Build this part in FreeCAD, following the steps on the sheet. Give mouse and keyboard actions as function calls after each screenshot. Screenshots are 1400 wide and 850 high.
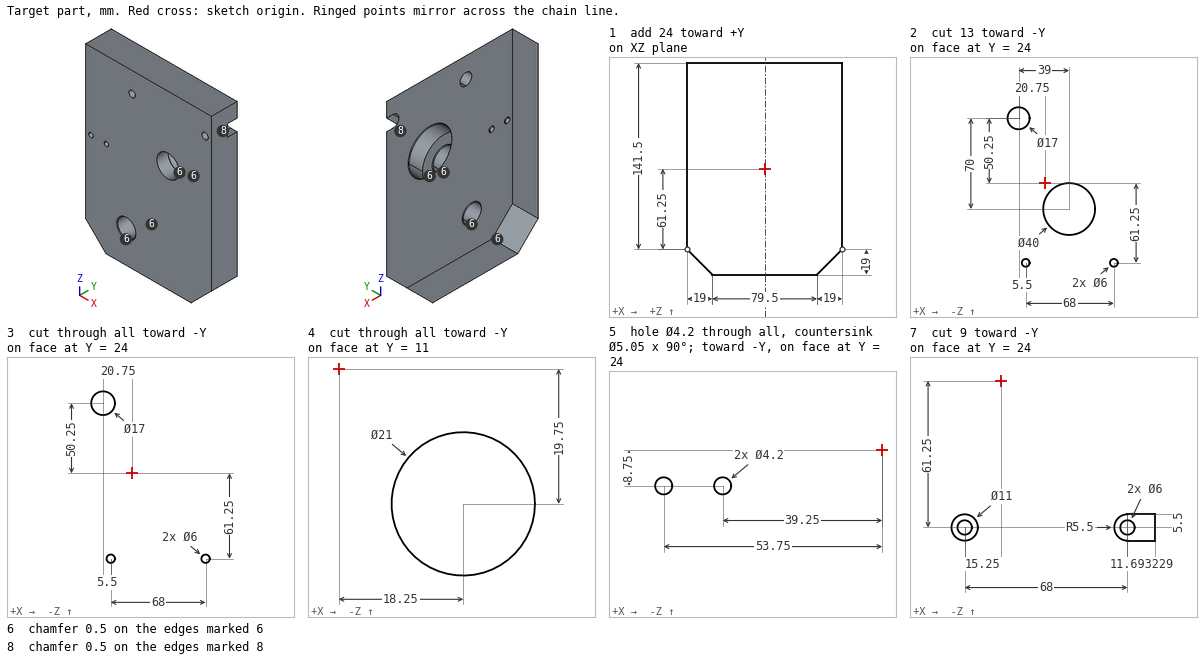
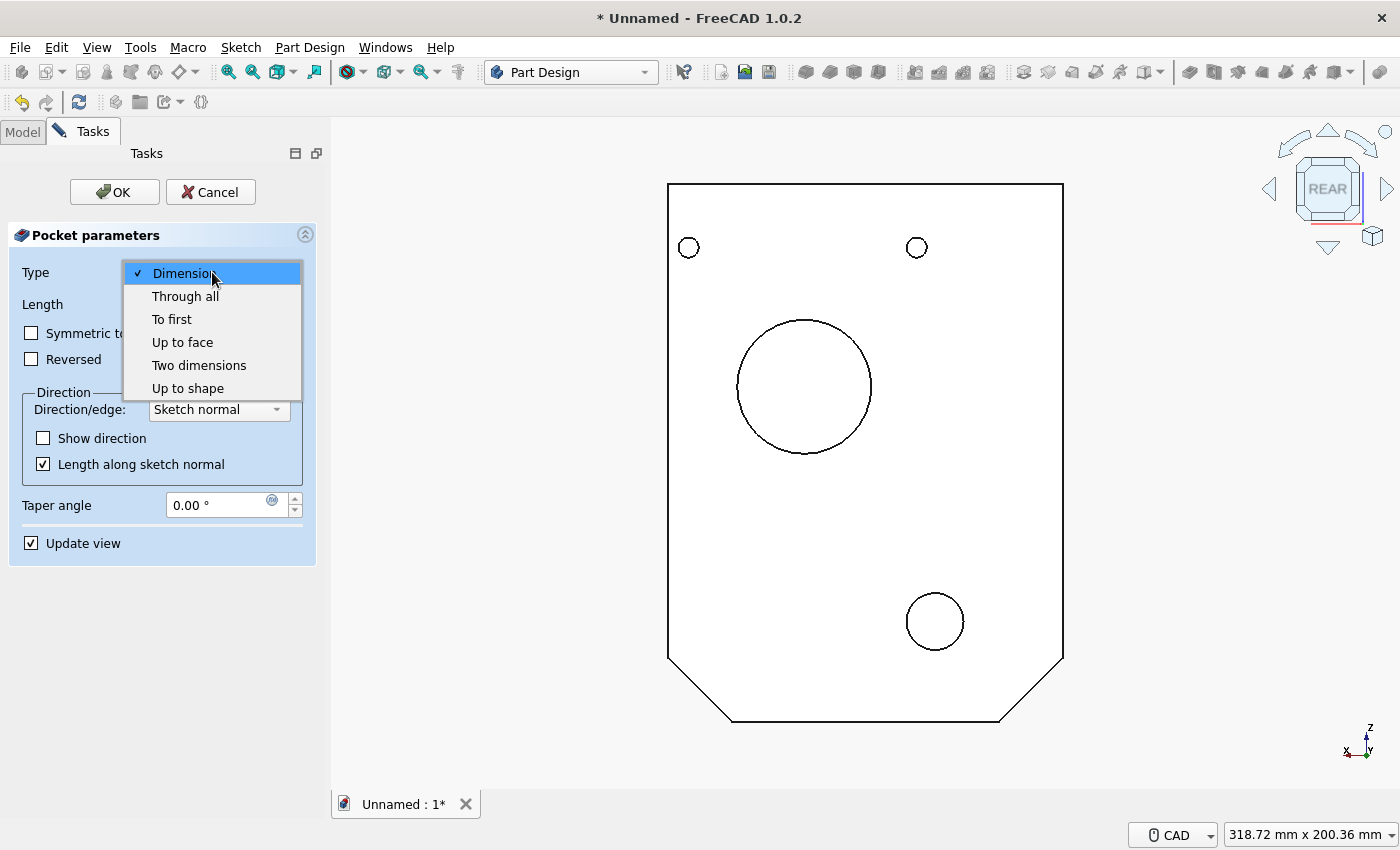
click(212, 296)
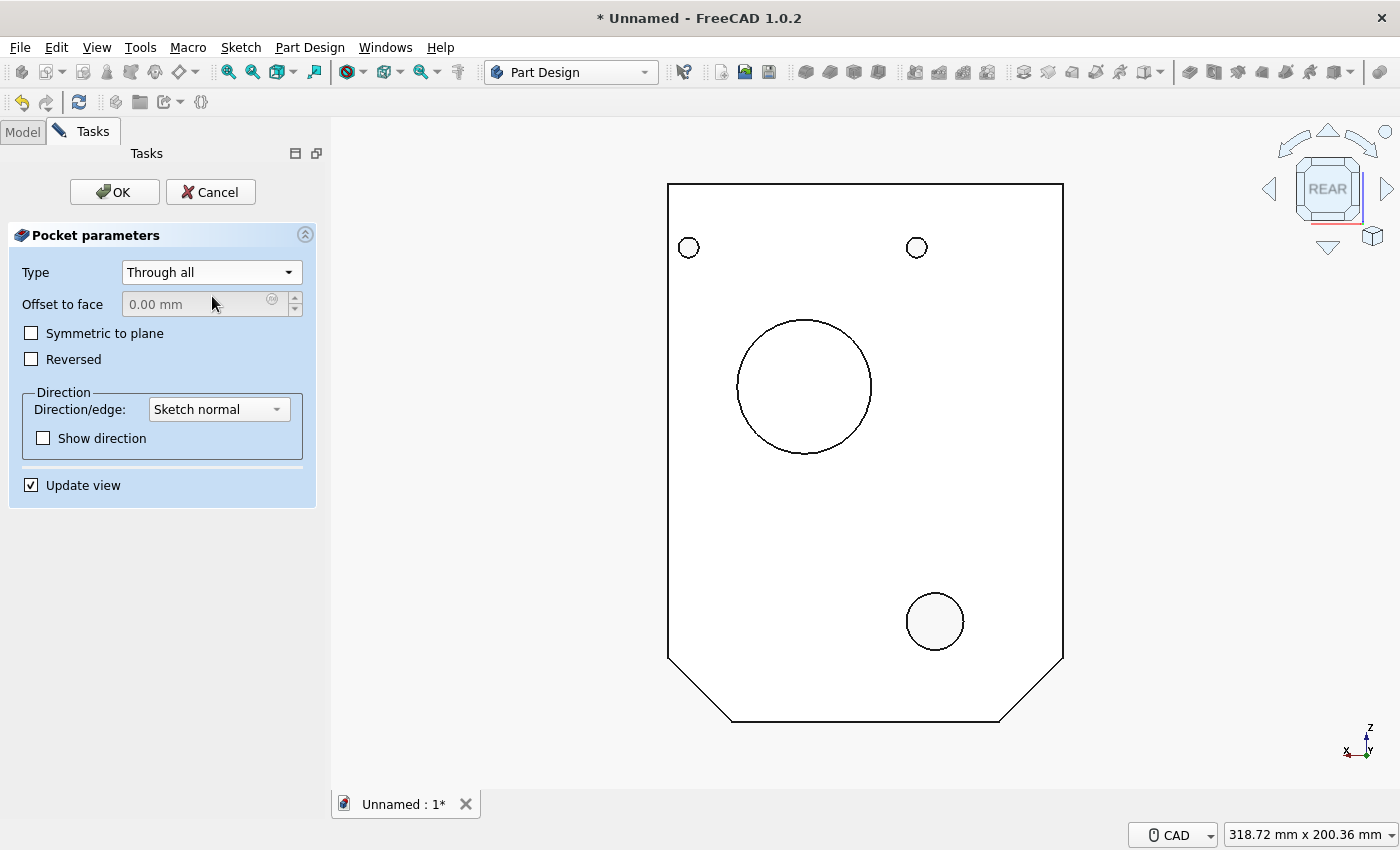
click(115, 192)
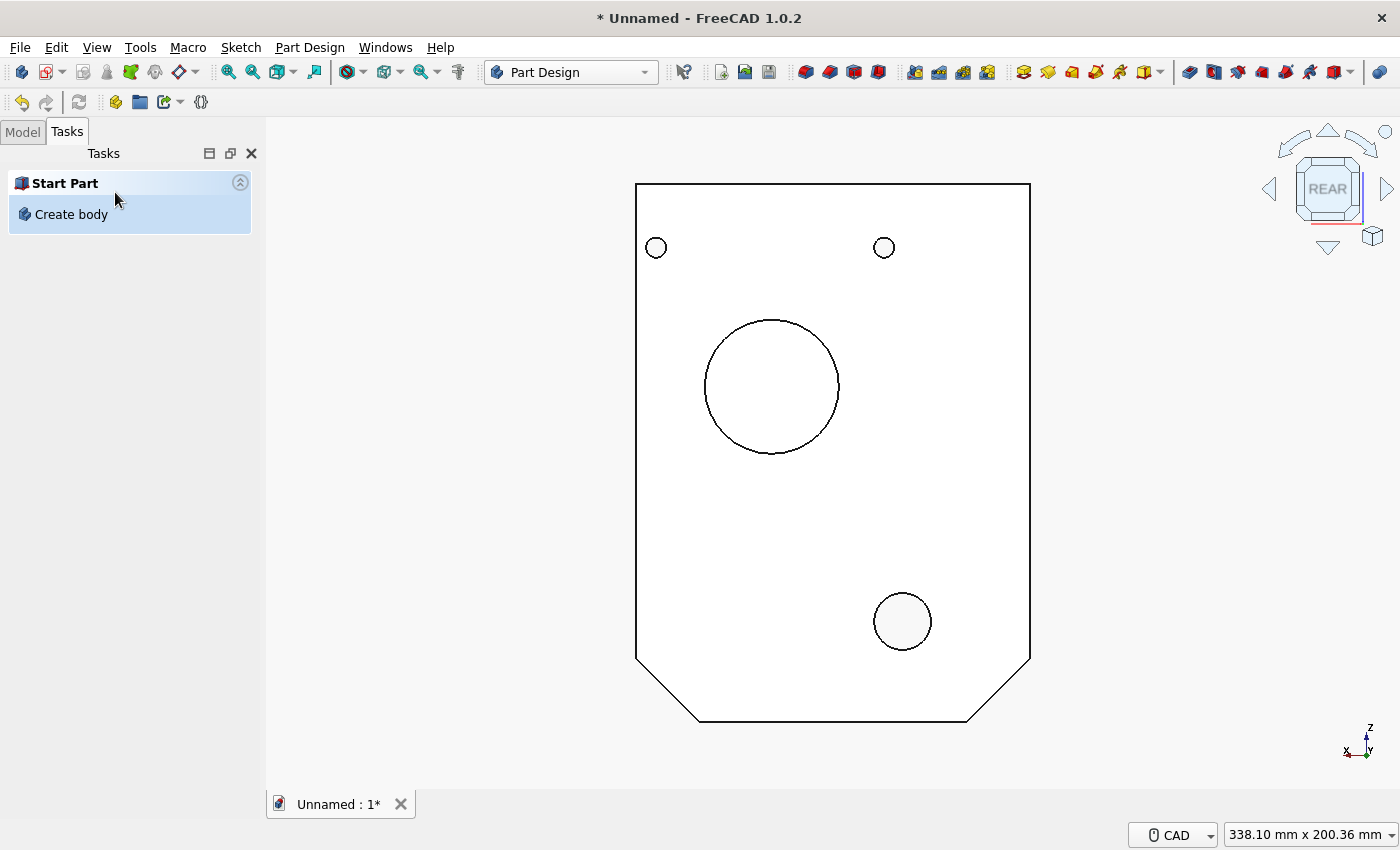
click(772, 386)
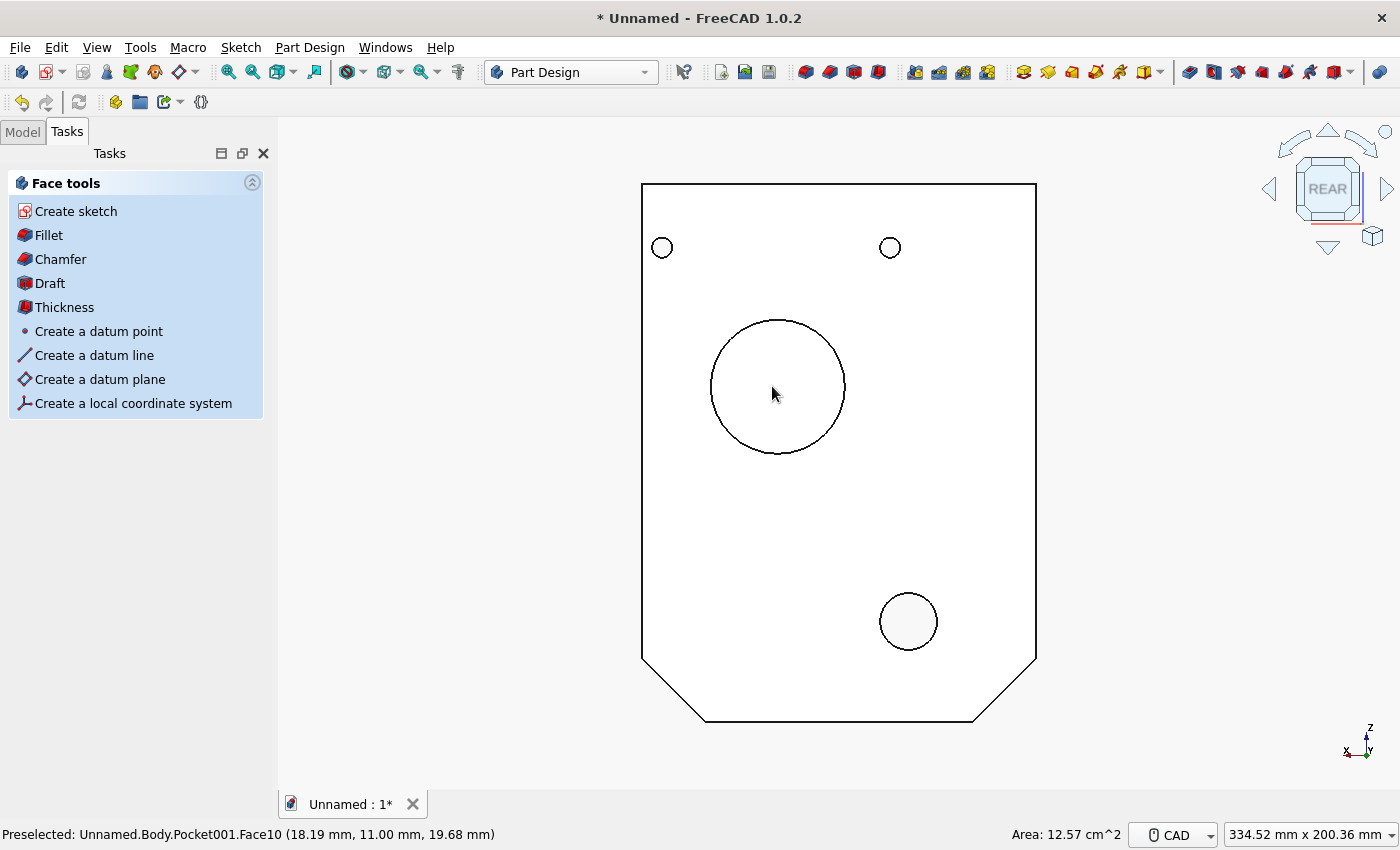
click(46, 72)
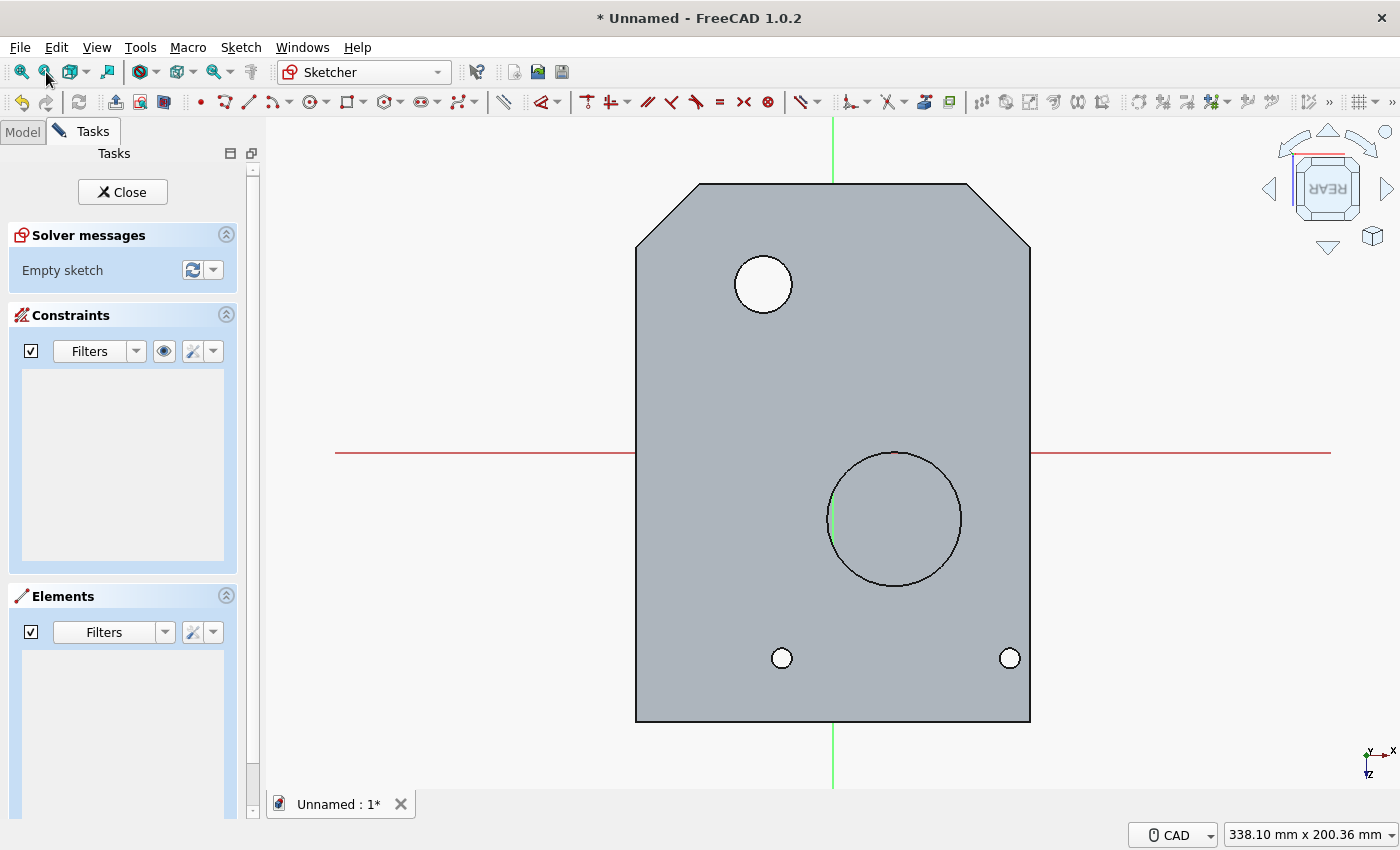
key(q)
key(s)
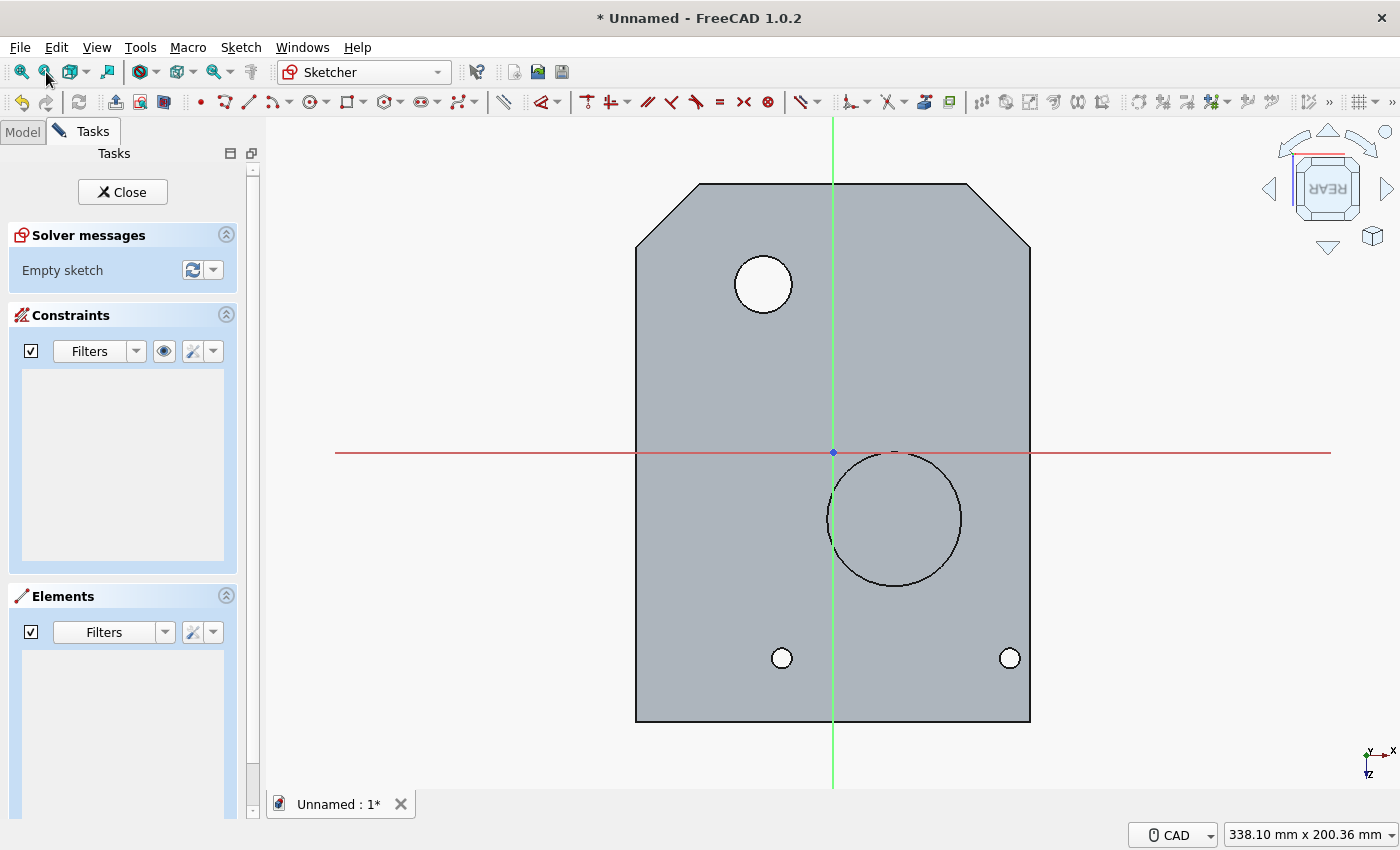
scroll(919, 520, up, 7)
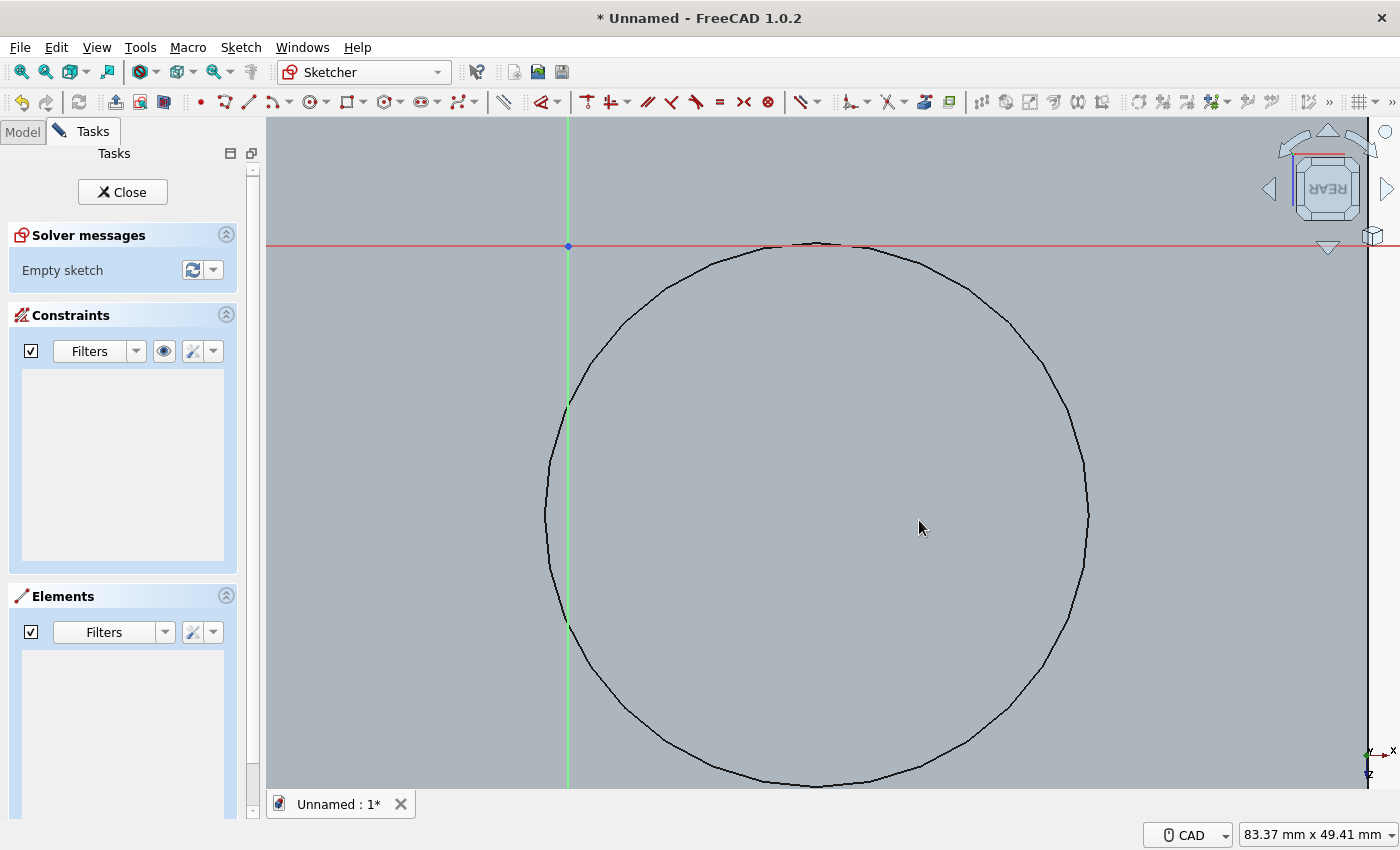
key(g)
key(c)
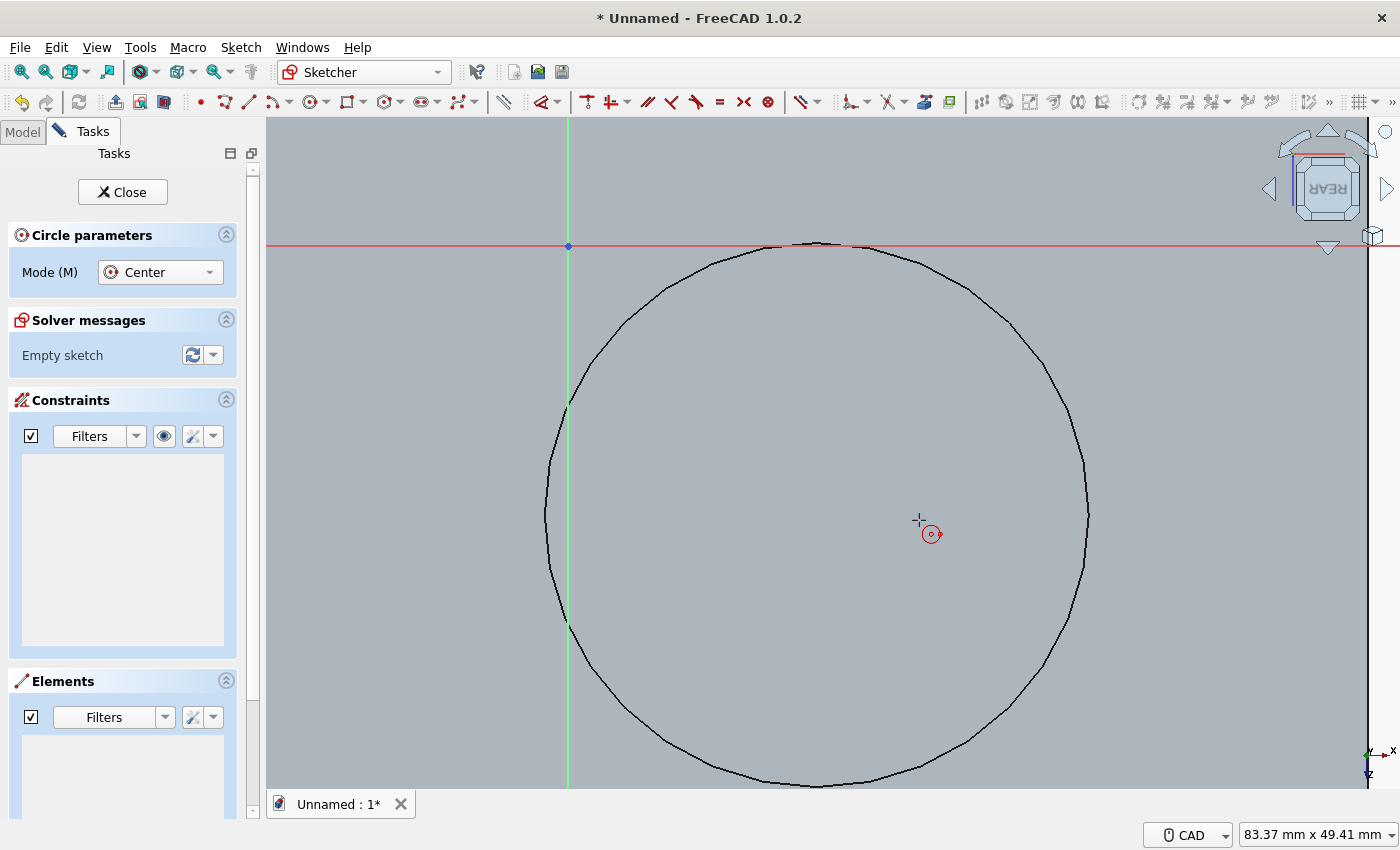
click(817, 515)
move(918, 414)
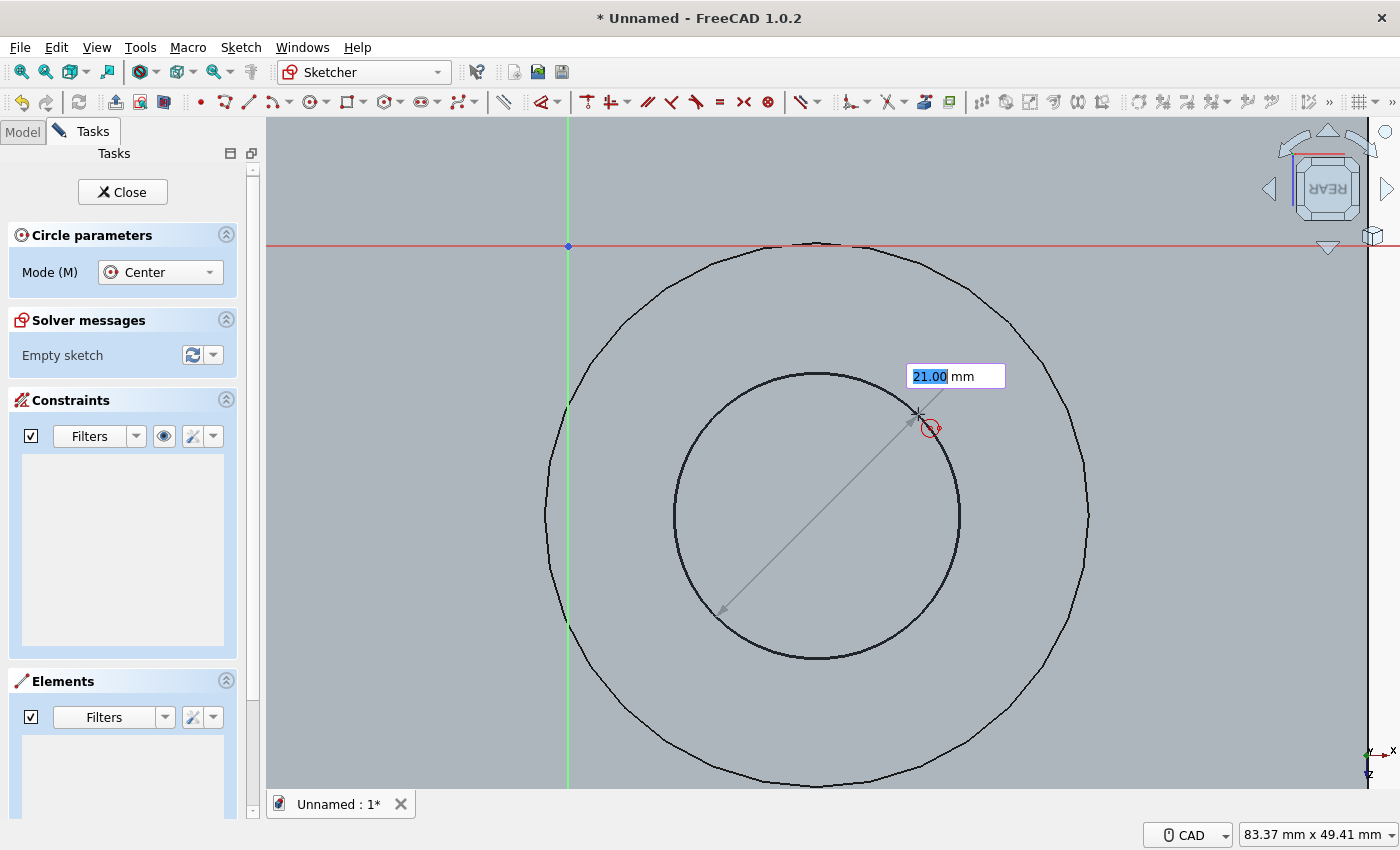
text(21)
key(Return)
key(Escape)